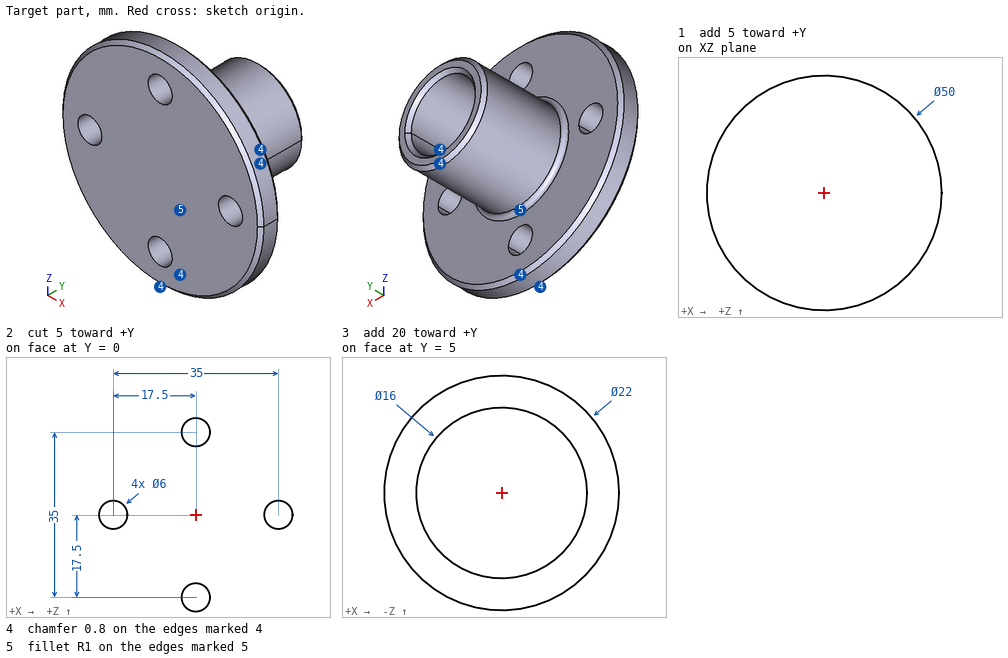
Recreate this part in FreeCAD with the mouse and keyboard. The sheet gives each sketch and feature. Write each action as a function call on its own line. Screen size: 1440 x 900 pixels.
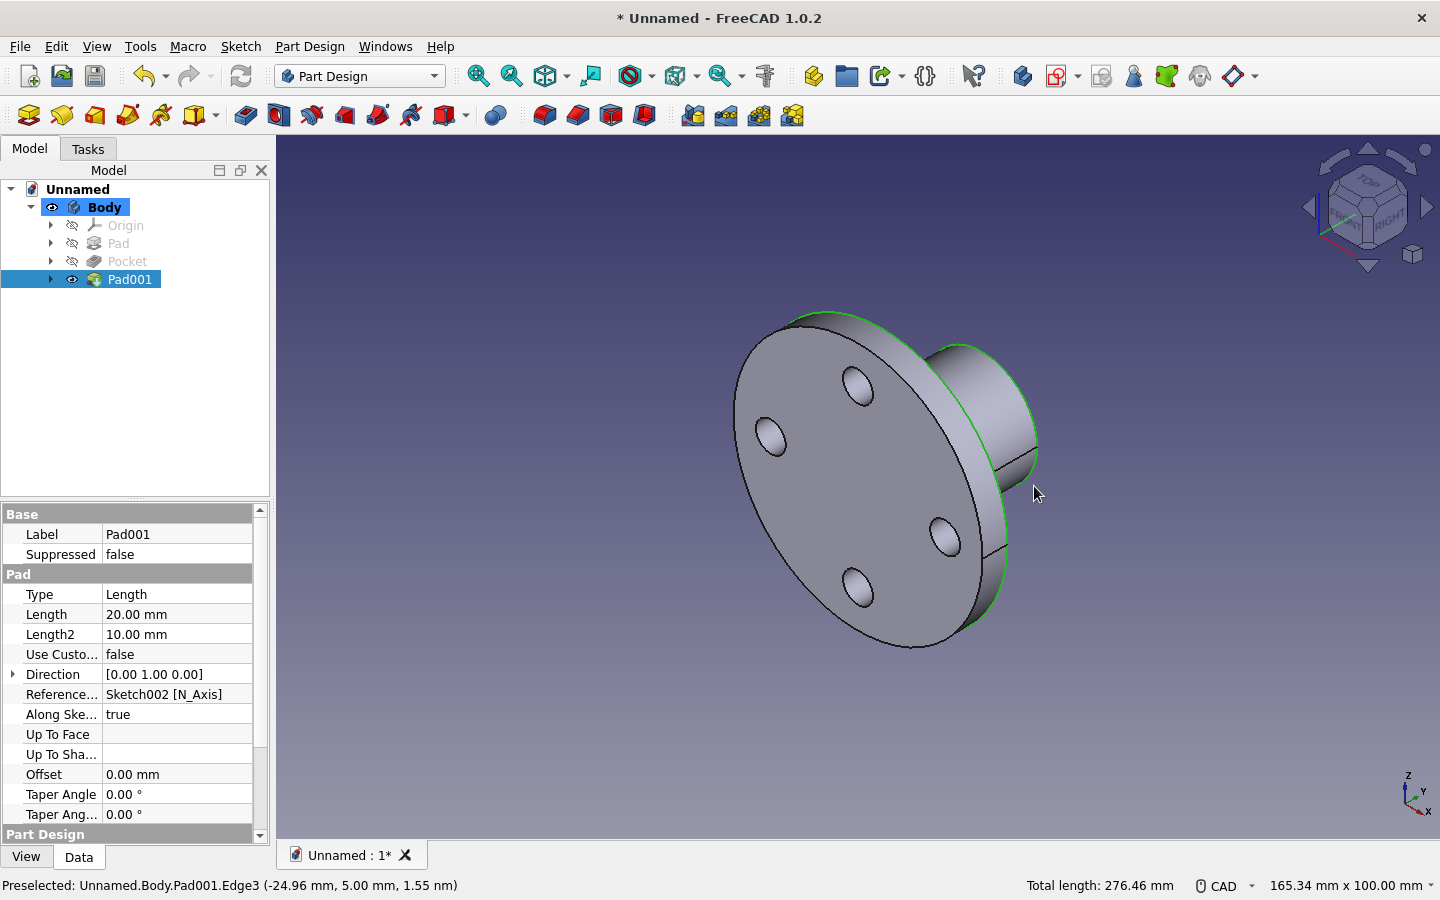
click(820, 327, ctrl)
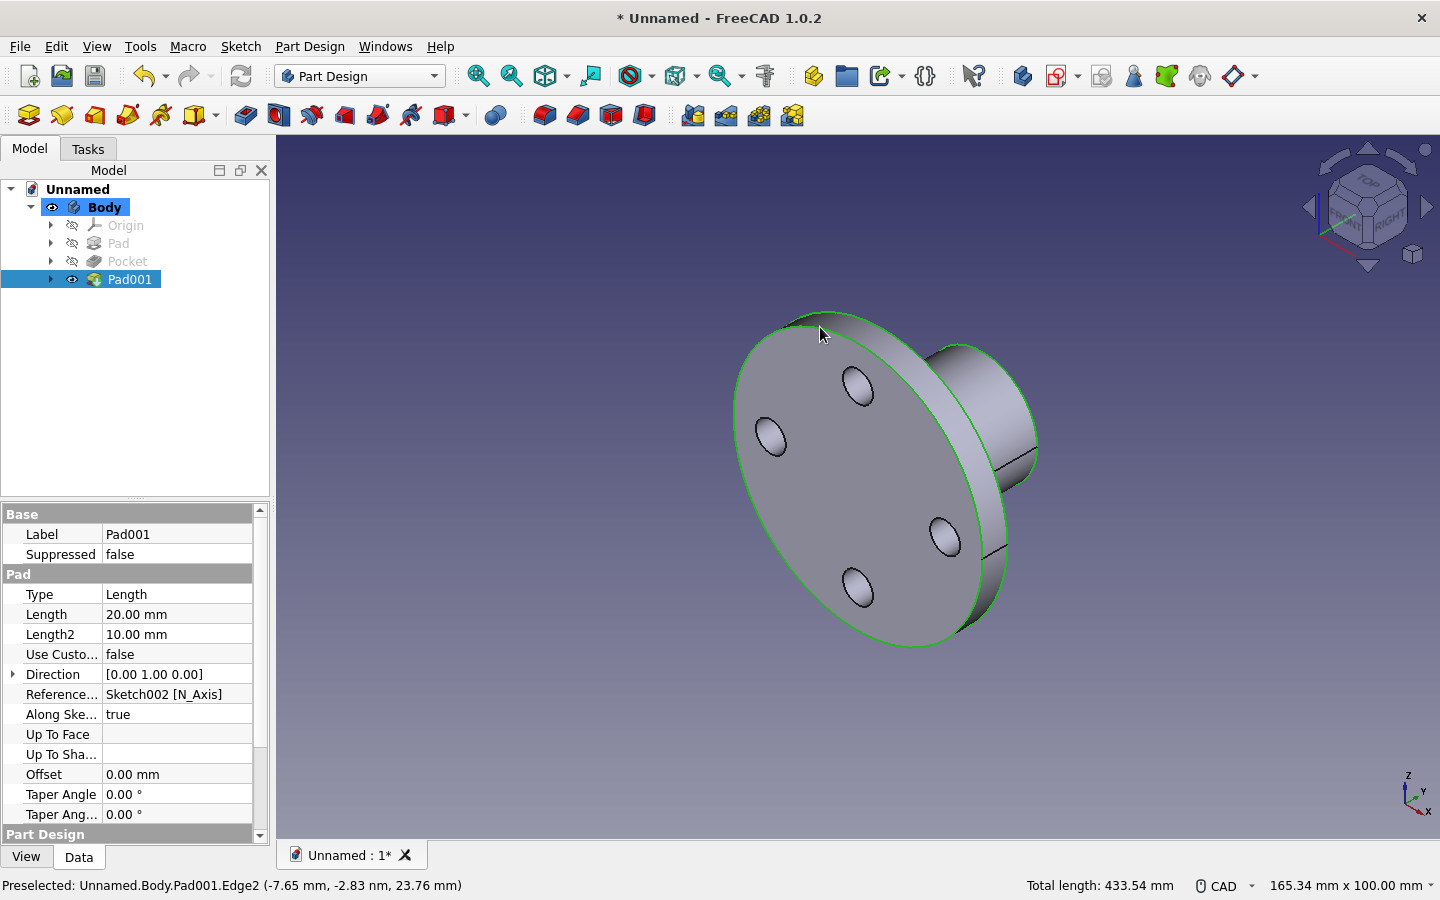
click(578, 116)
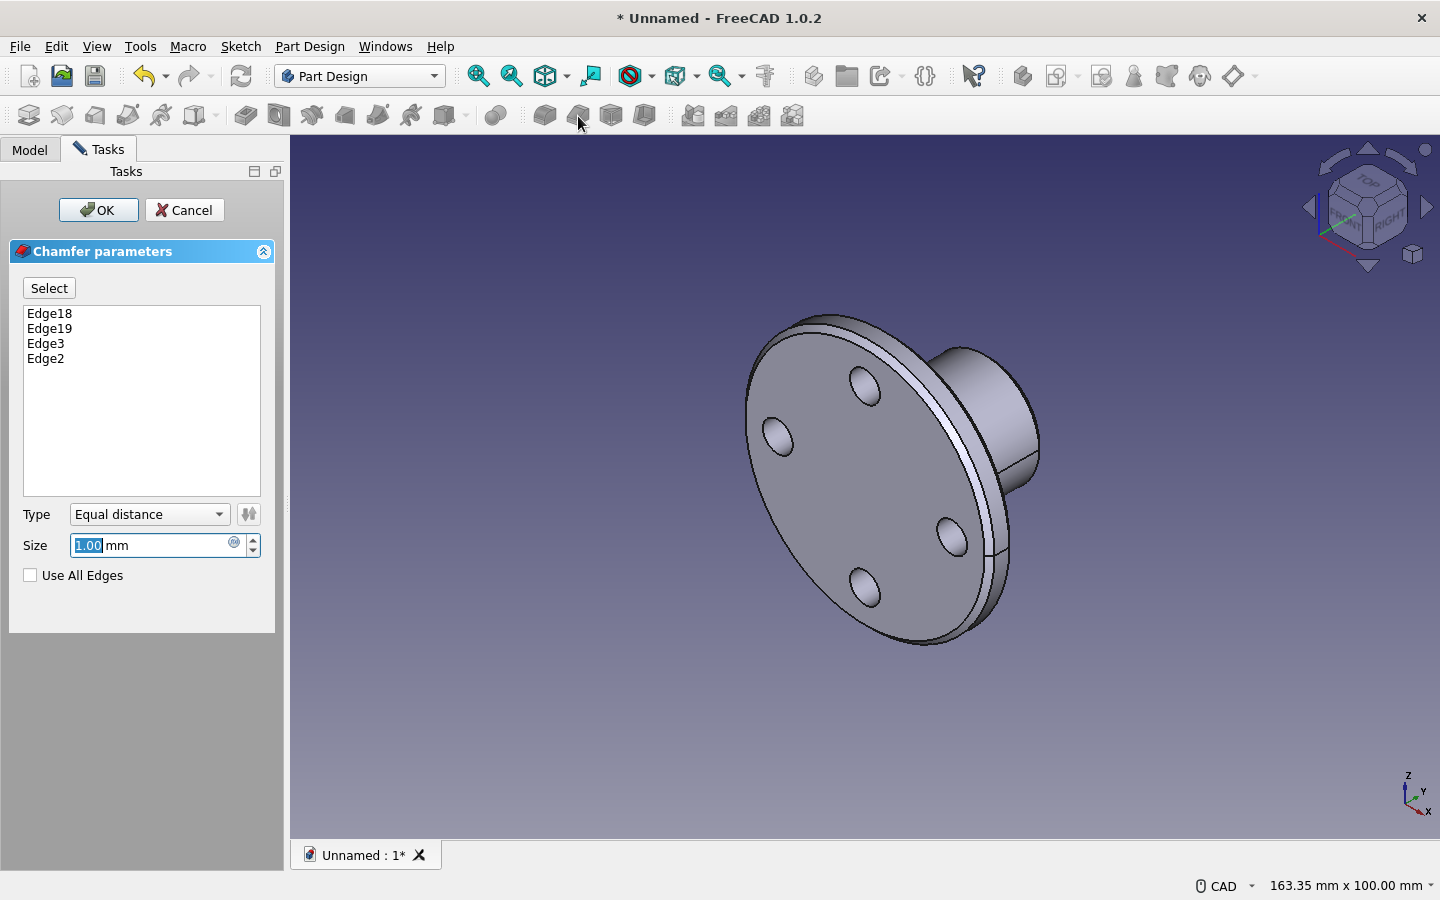
text(0.8)
key(Tab)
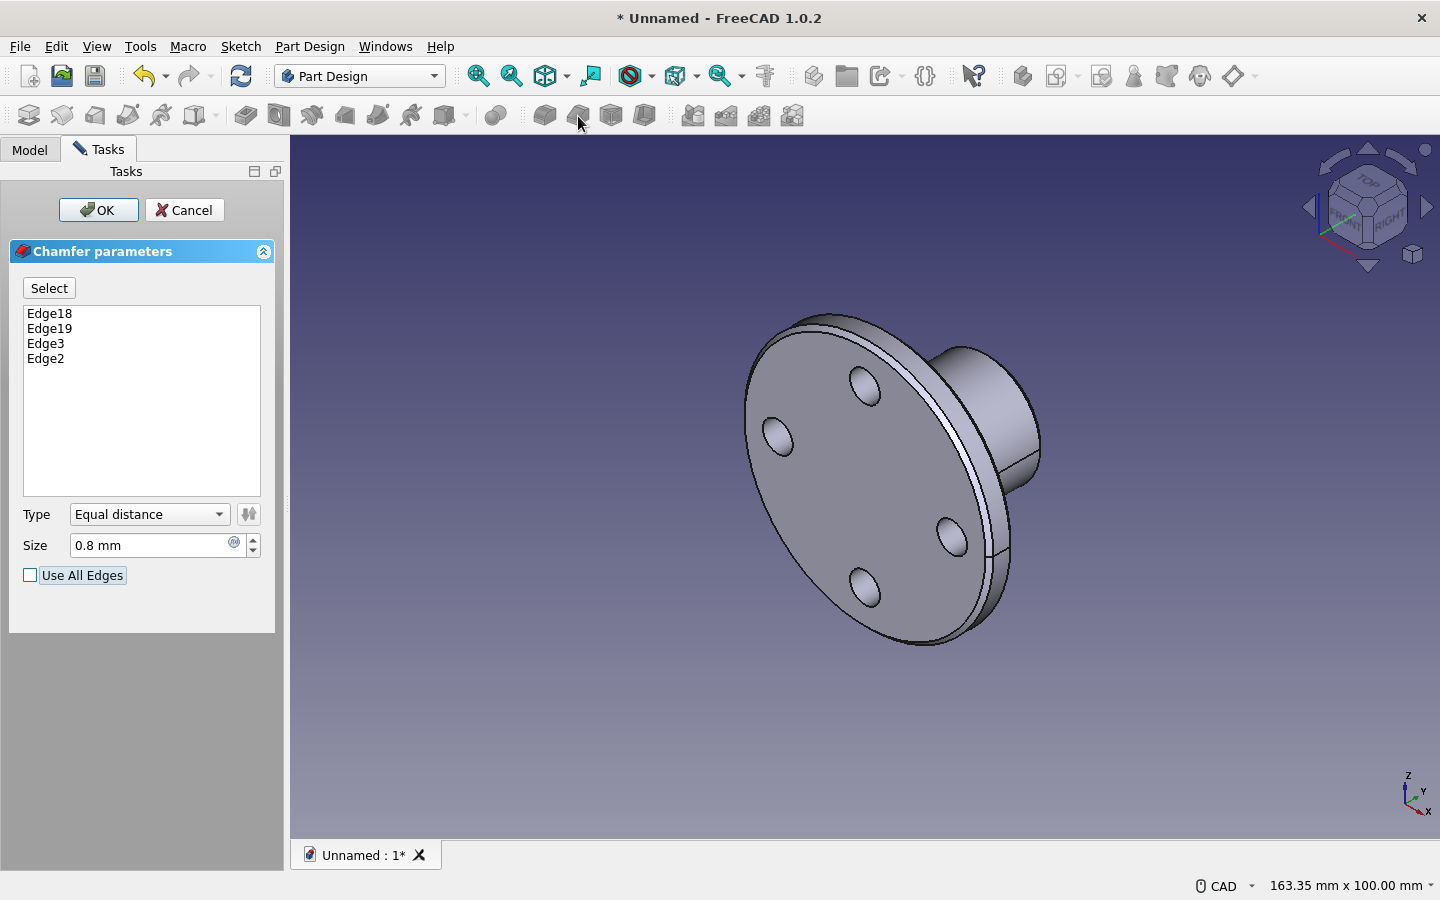
click(99, 210)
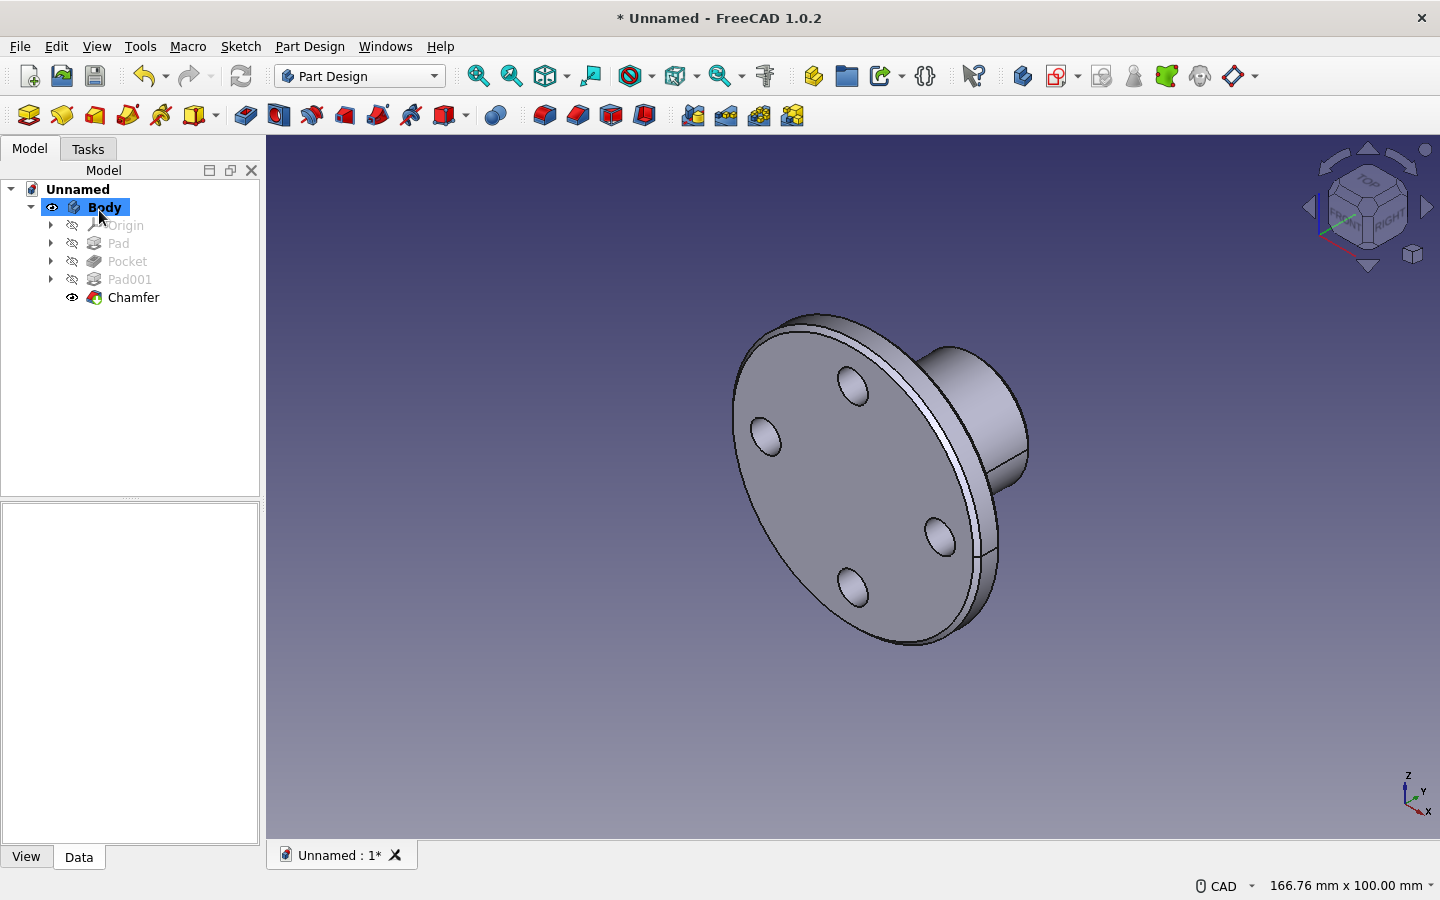
key(2)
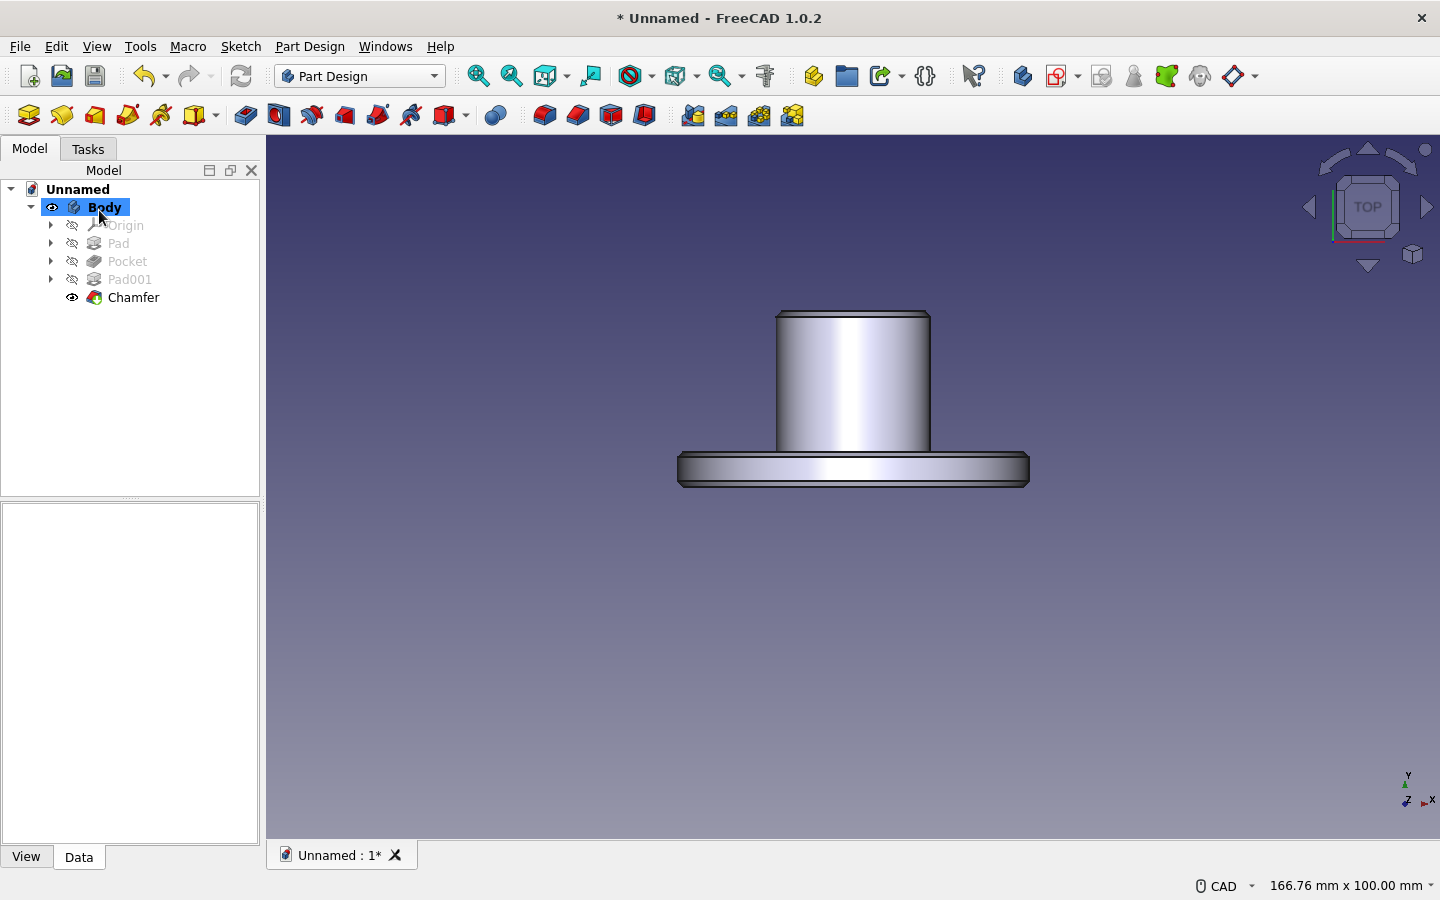
click(479, 76)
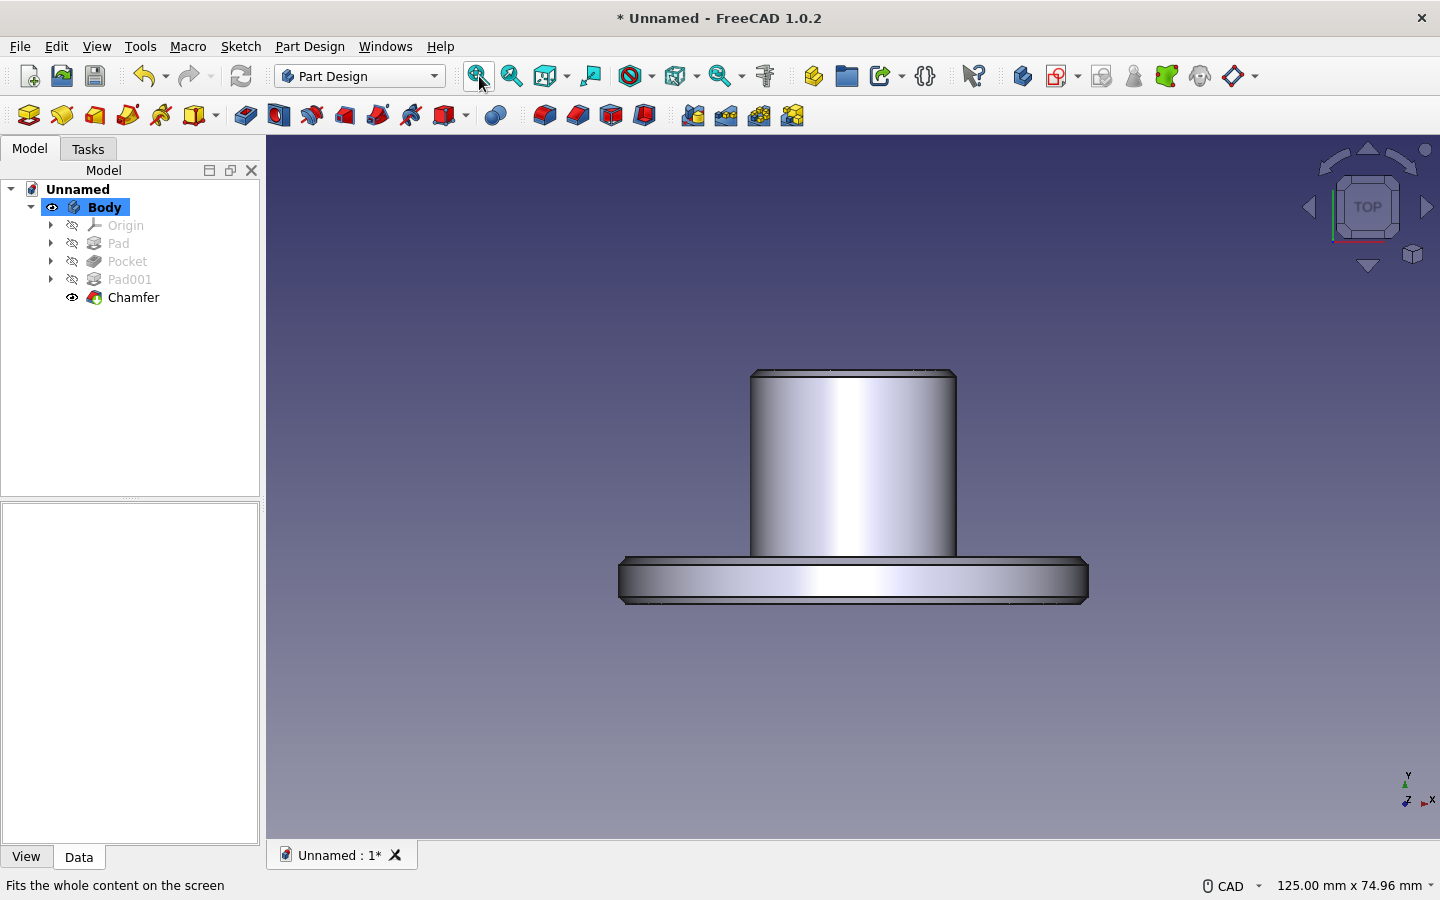
key(0)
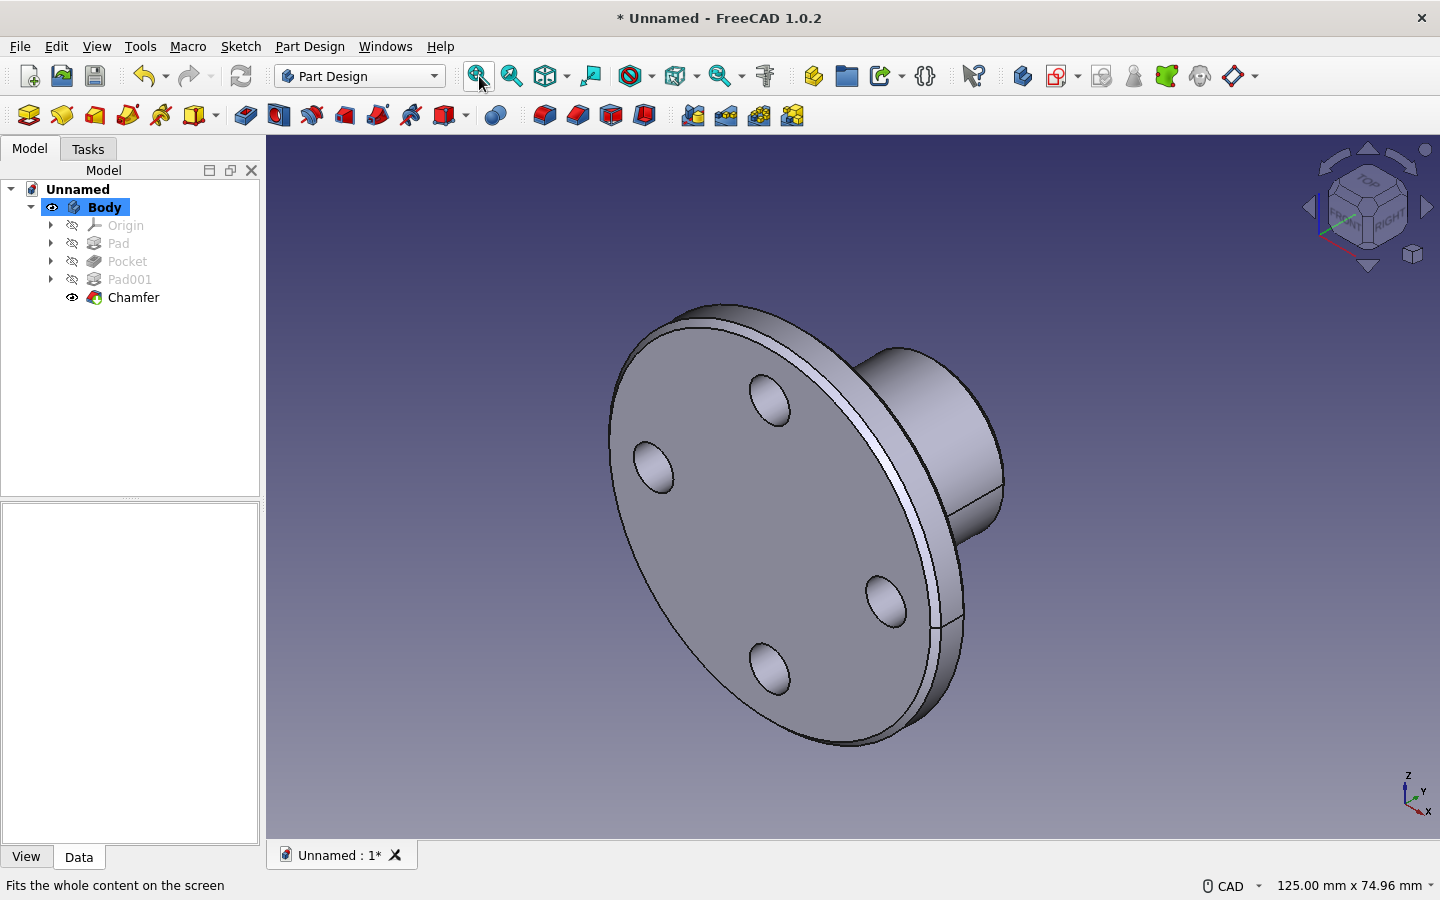
key(1)